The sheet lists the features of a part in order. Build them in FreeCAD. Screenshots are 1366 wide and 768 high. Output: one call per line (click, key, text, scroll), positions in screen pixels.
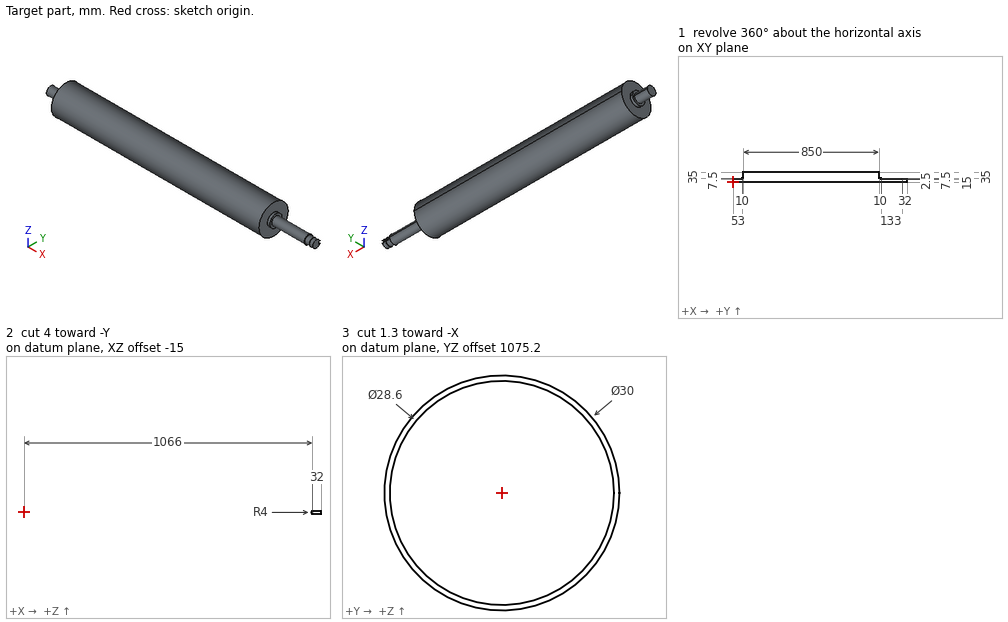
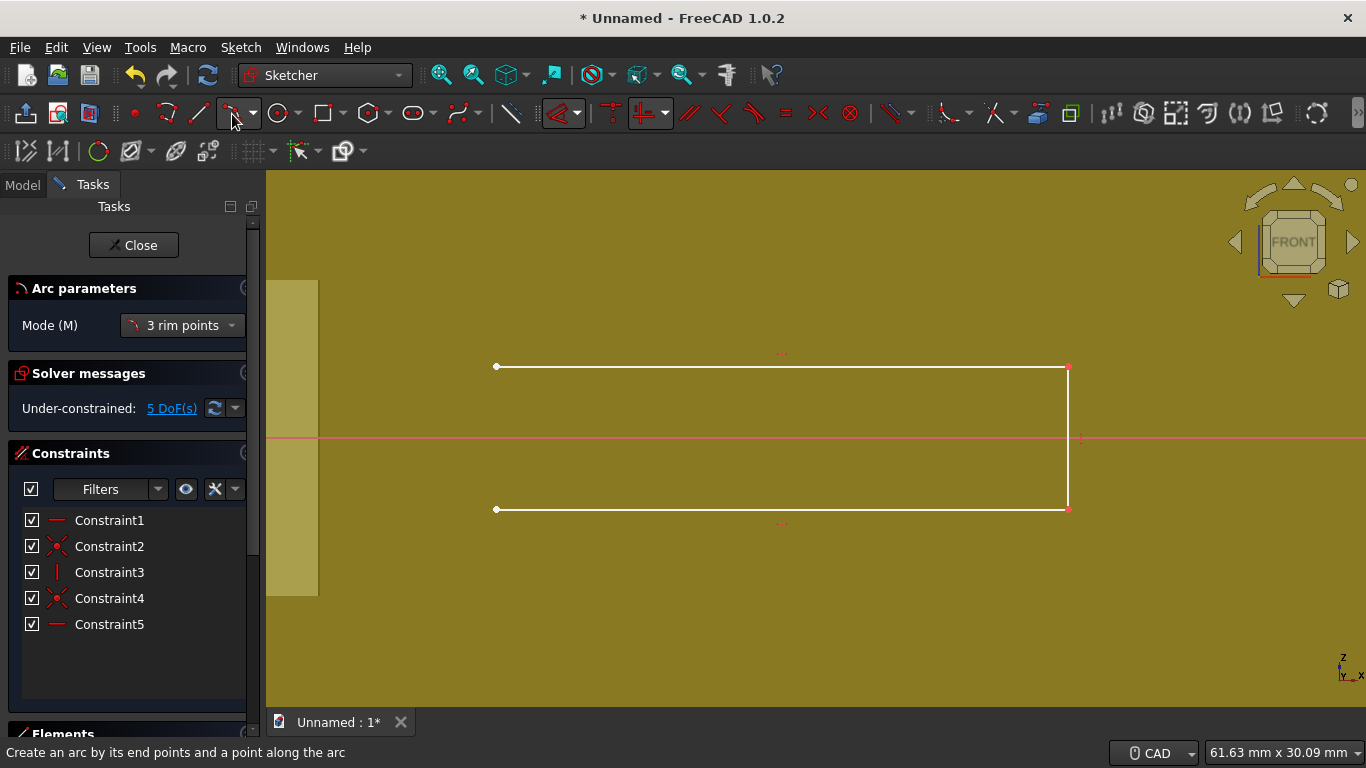
click(497, 510)
click(497, 367)
click(429, 416)
key(Escape)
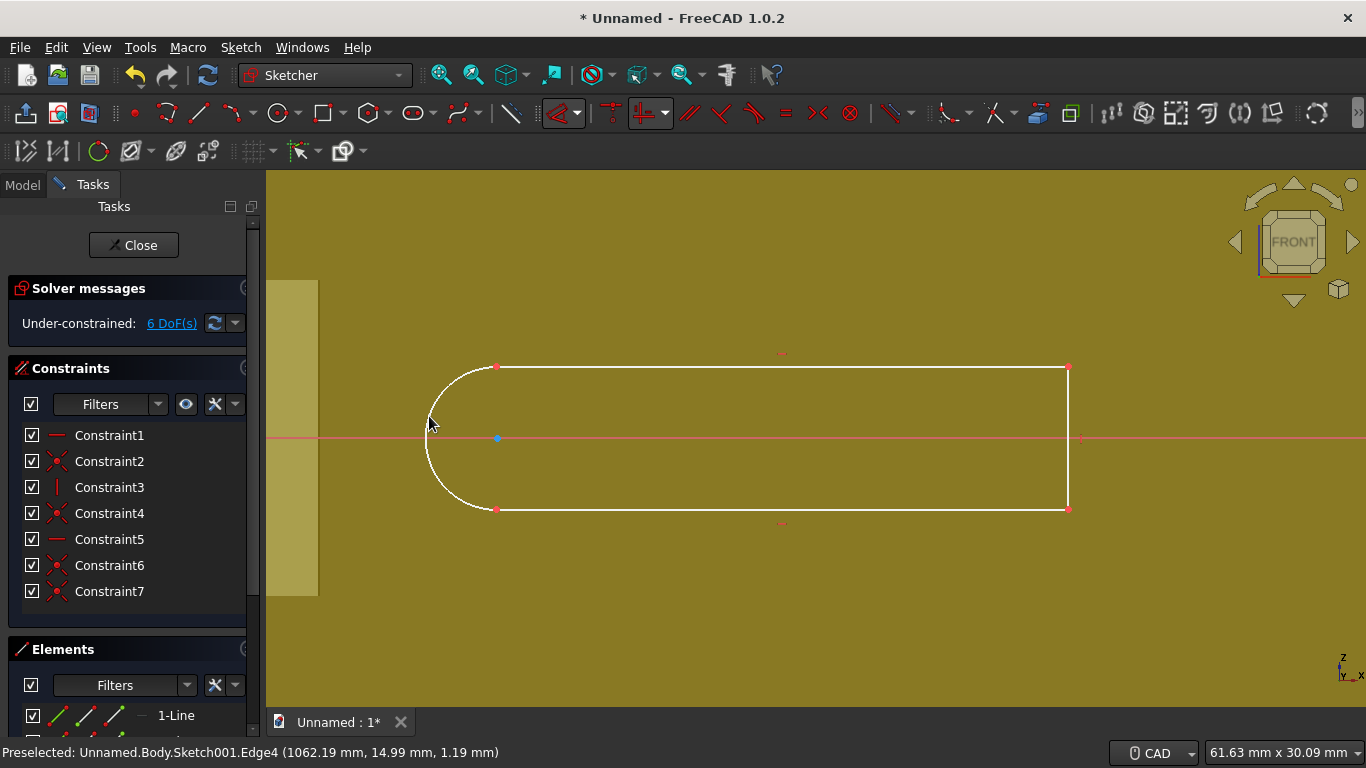
click(668, 367)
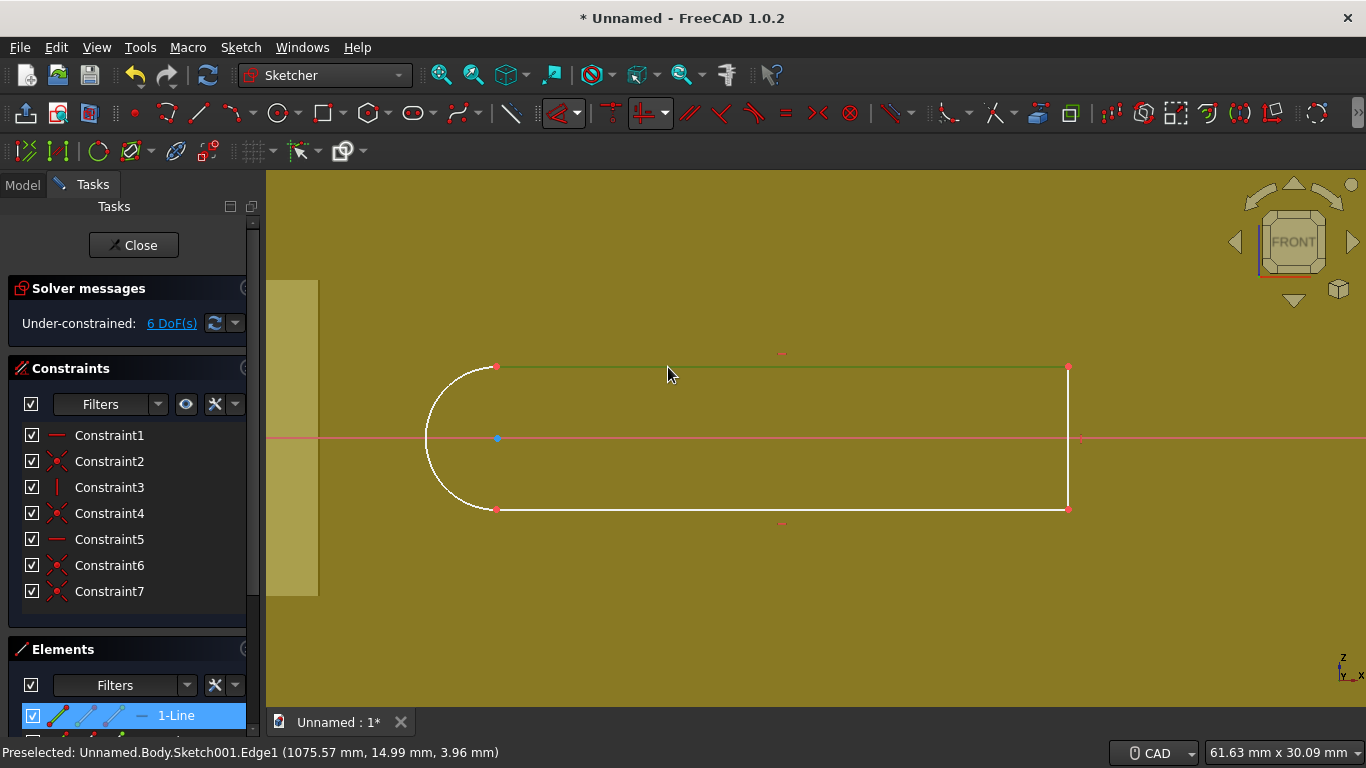
click(439, 397)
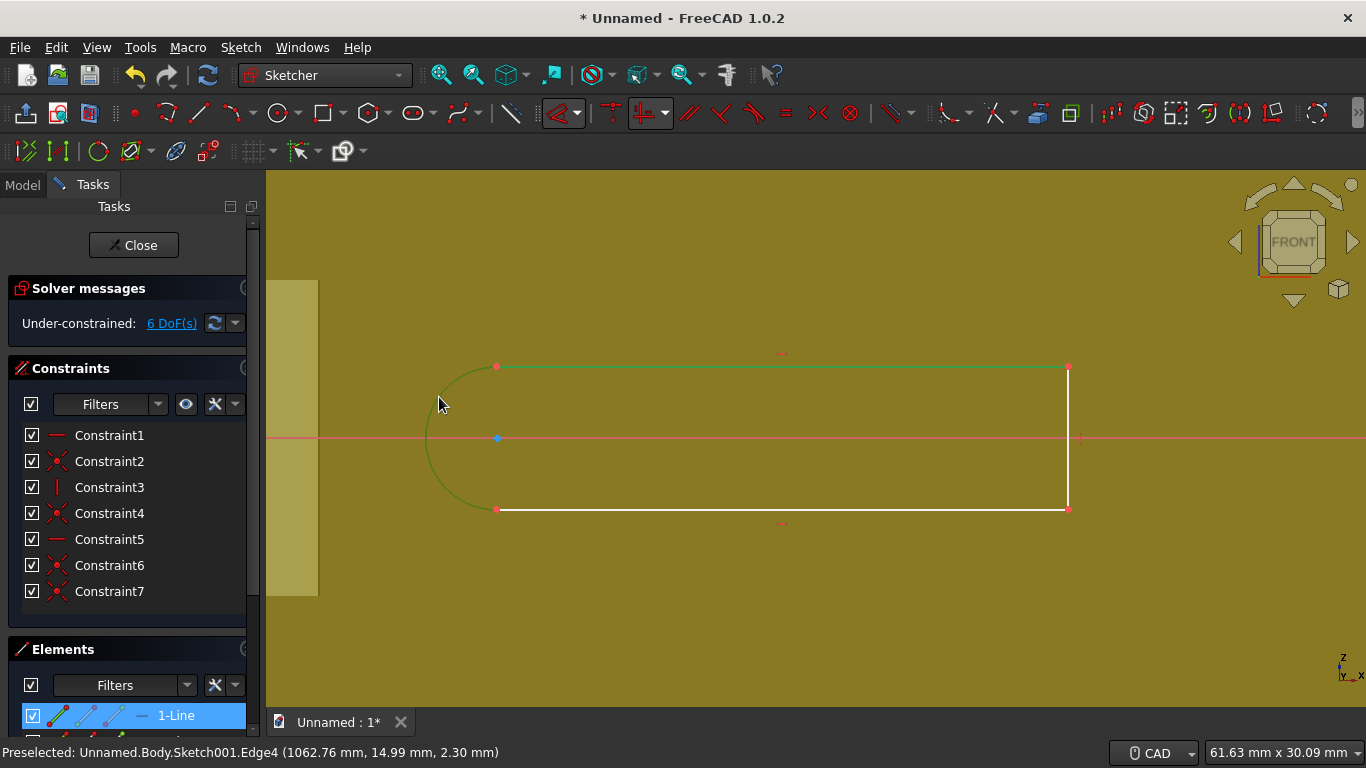
click(754, 114)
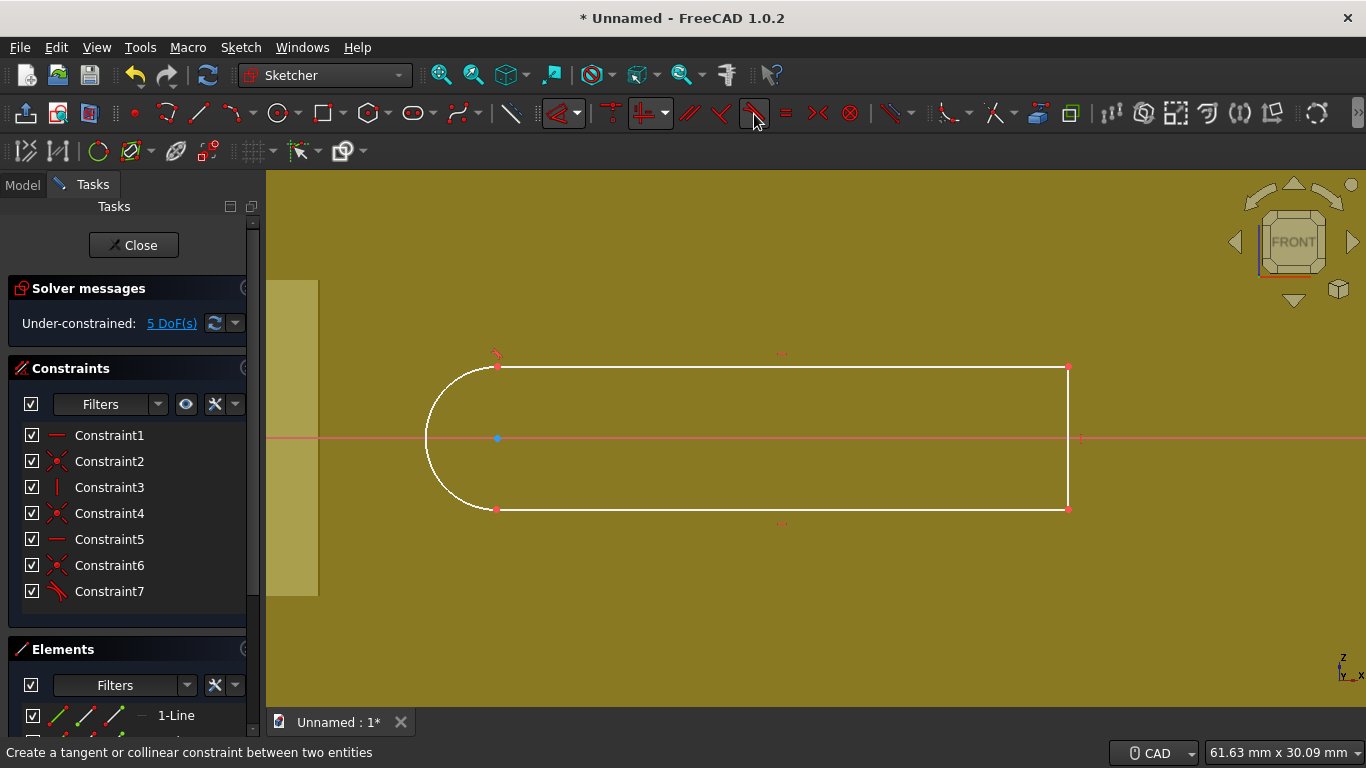
click(897, 510)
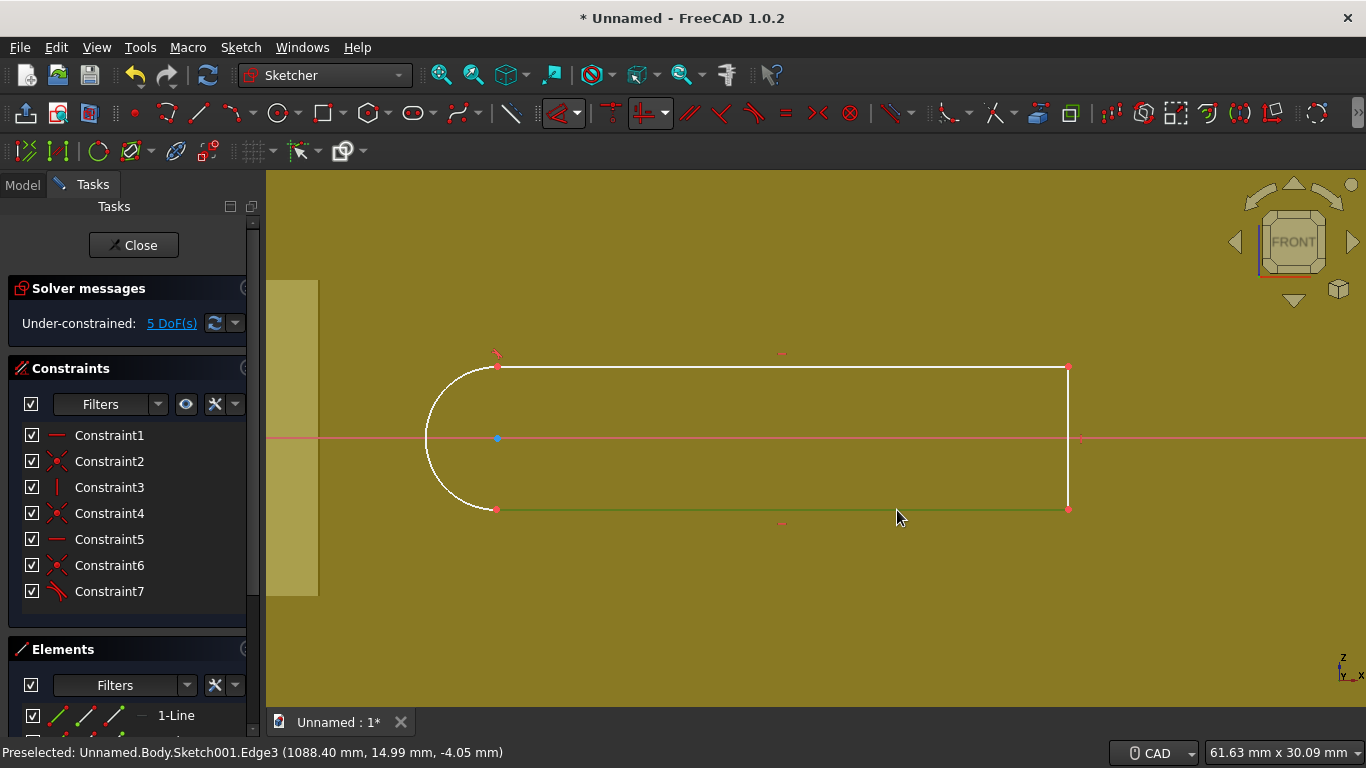
click(439, 396)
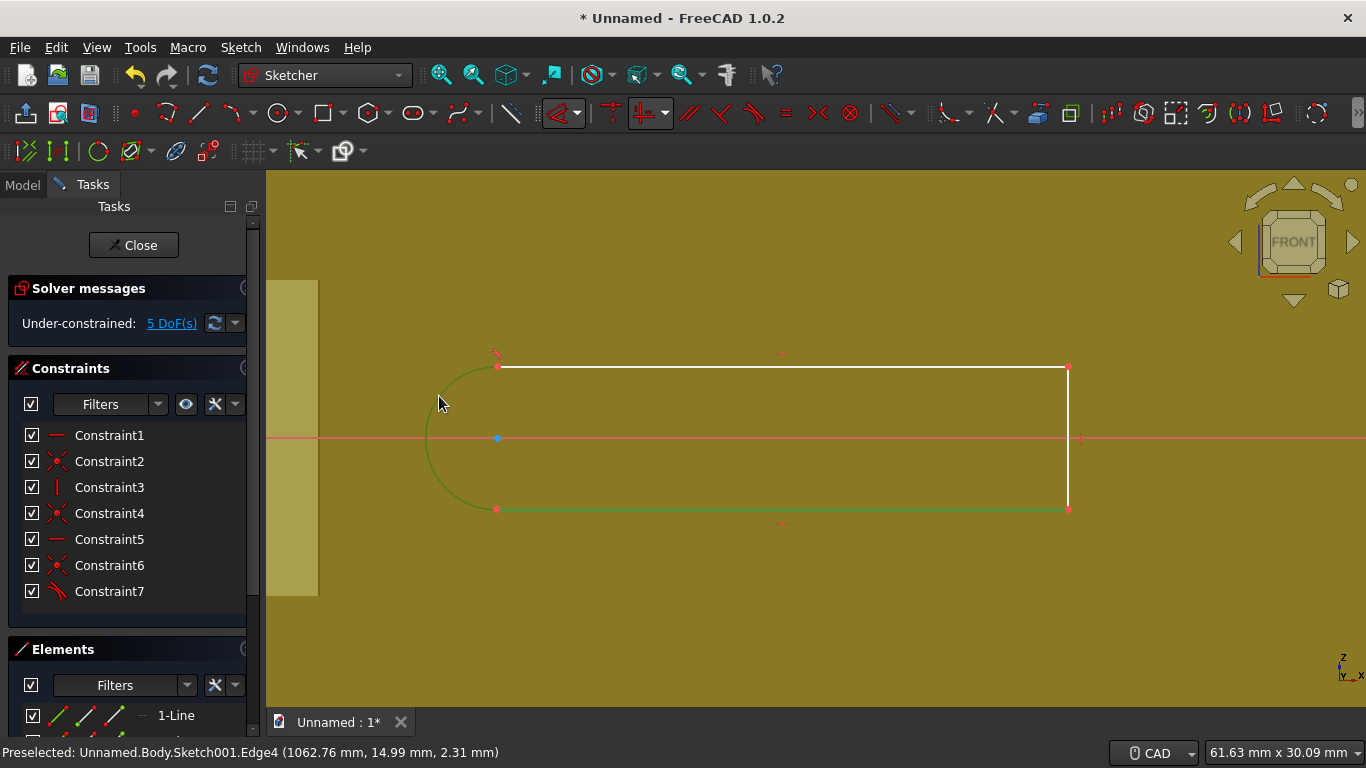
key(t)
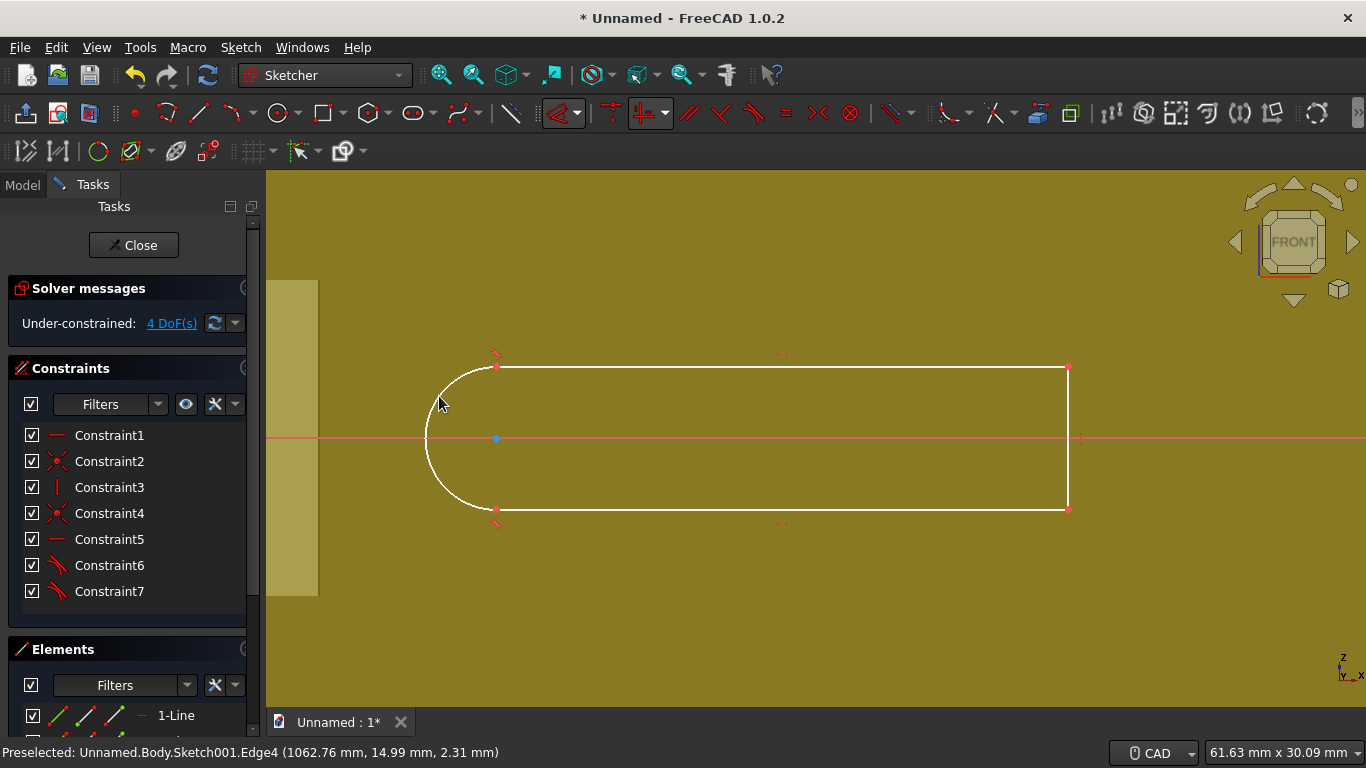
click(497, 438)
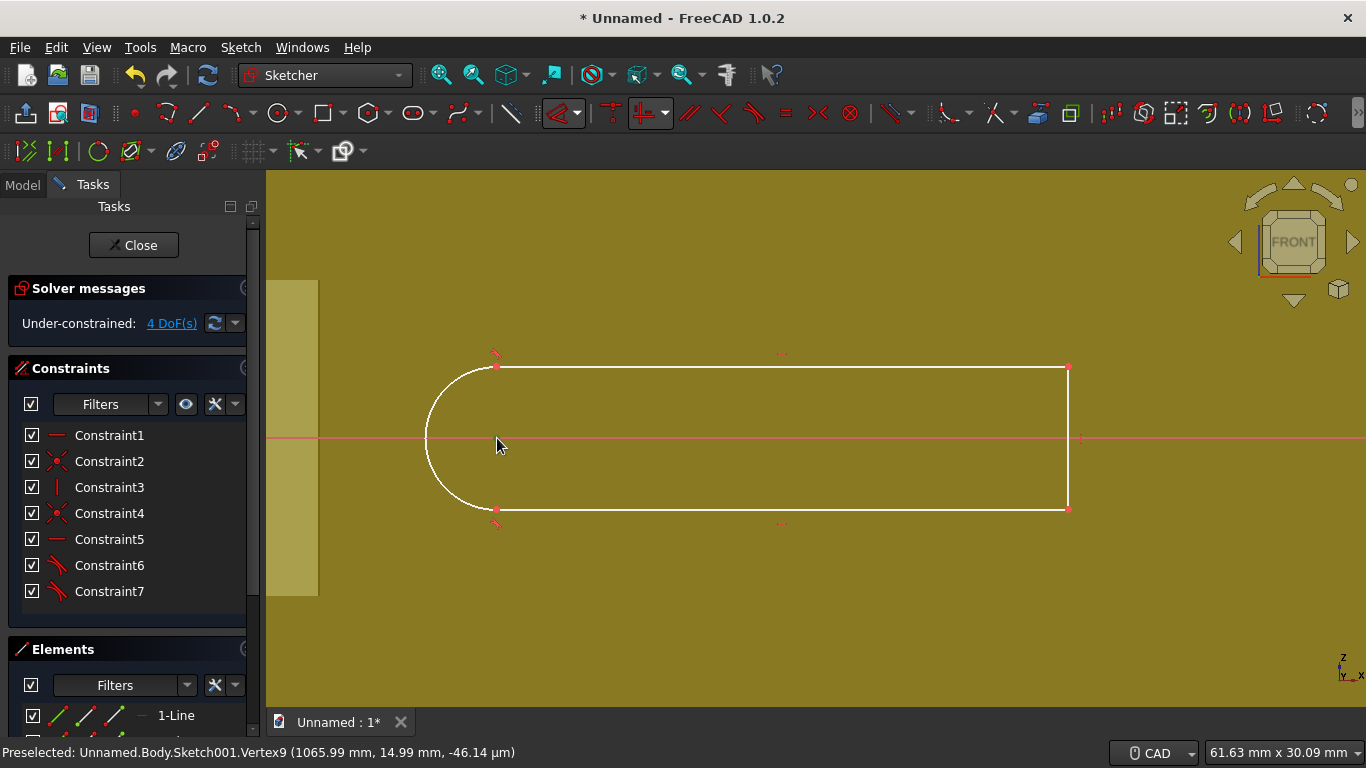
click(359, 438)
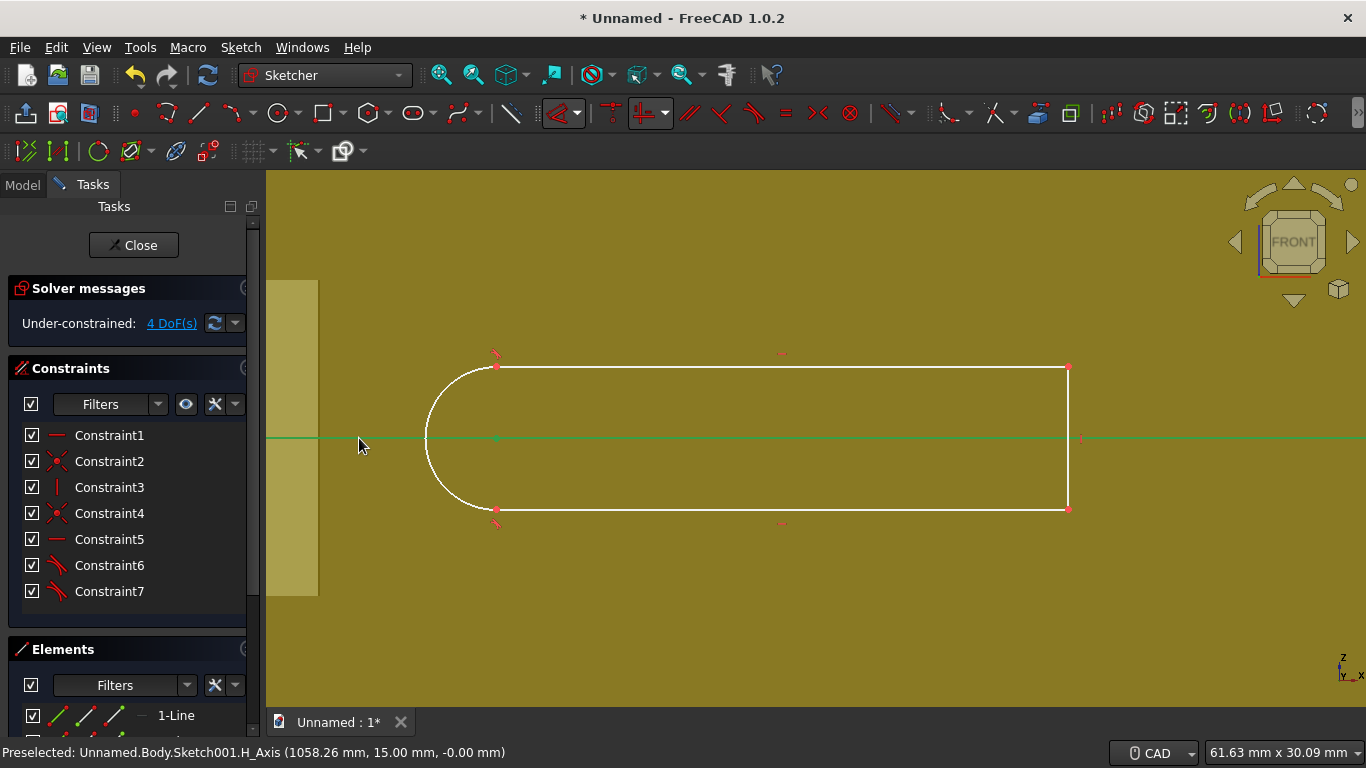
click(612, 114)